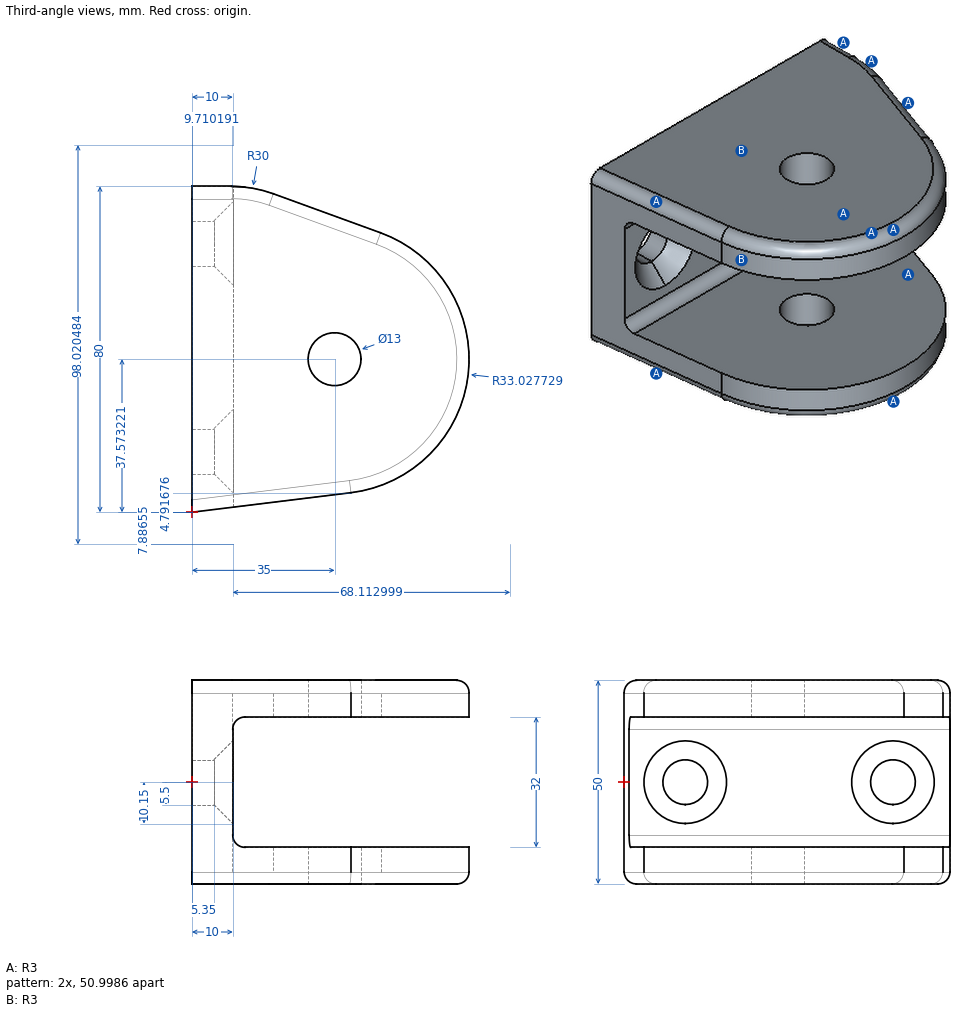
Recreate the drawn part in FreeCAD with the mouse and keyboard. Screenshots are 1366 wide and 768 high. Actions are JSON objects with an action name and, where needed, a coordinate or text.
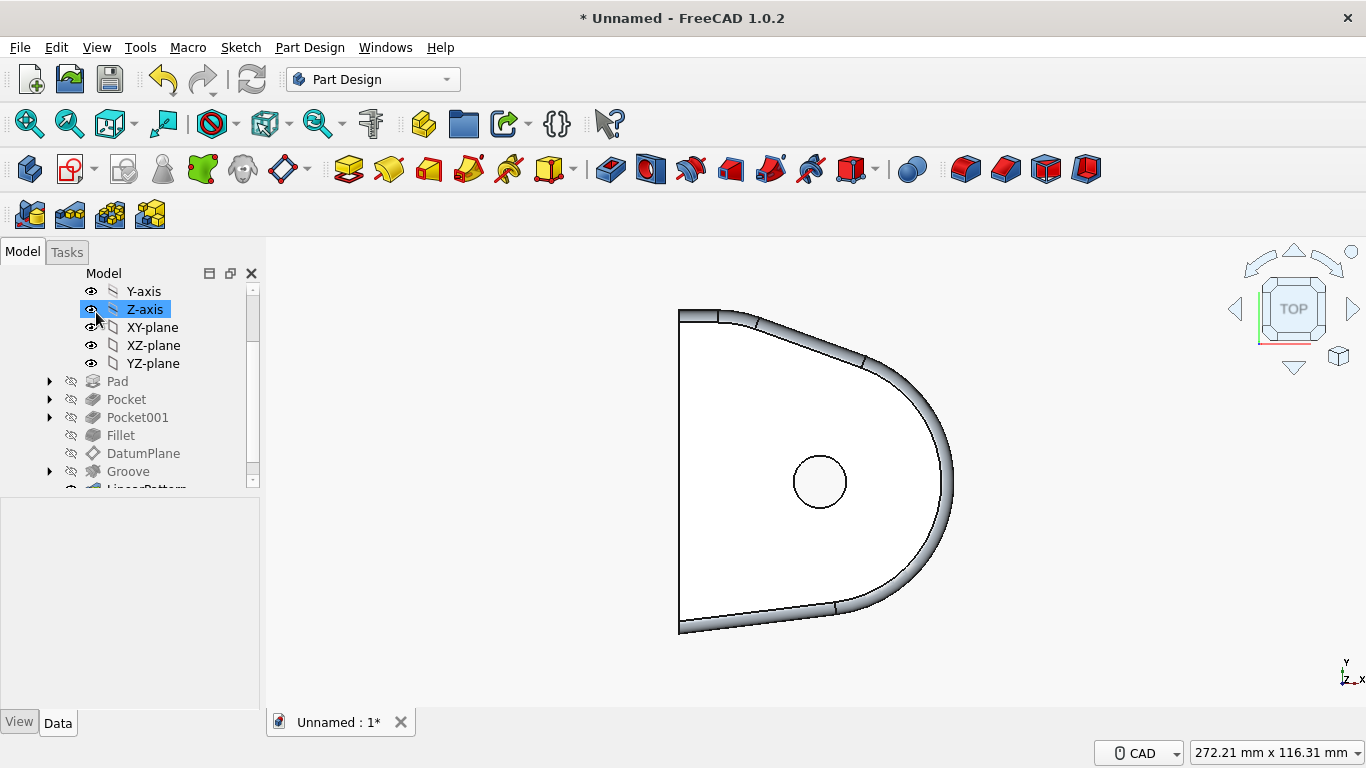
{"action": "key", "text": "1"}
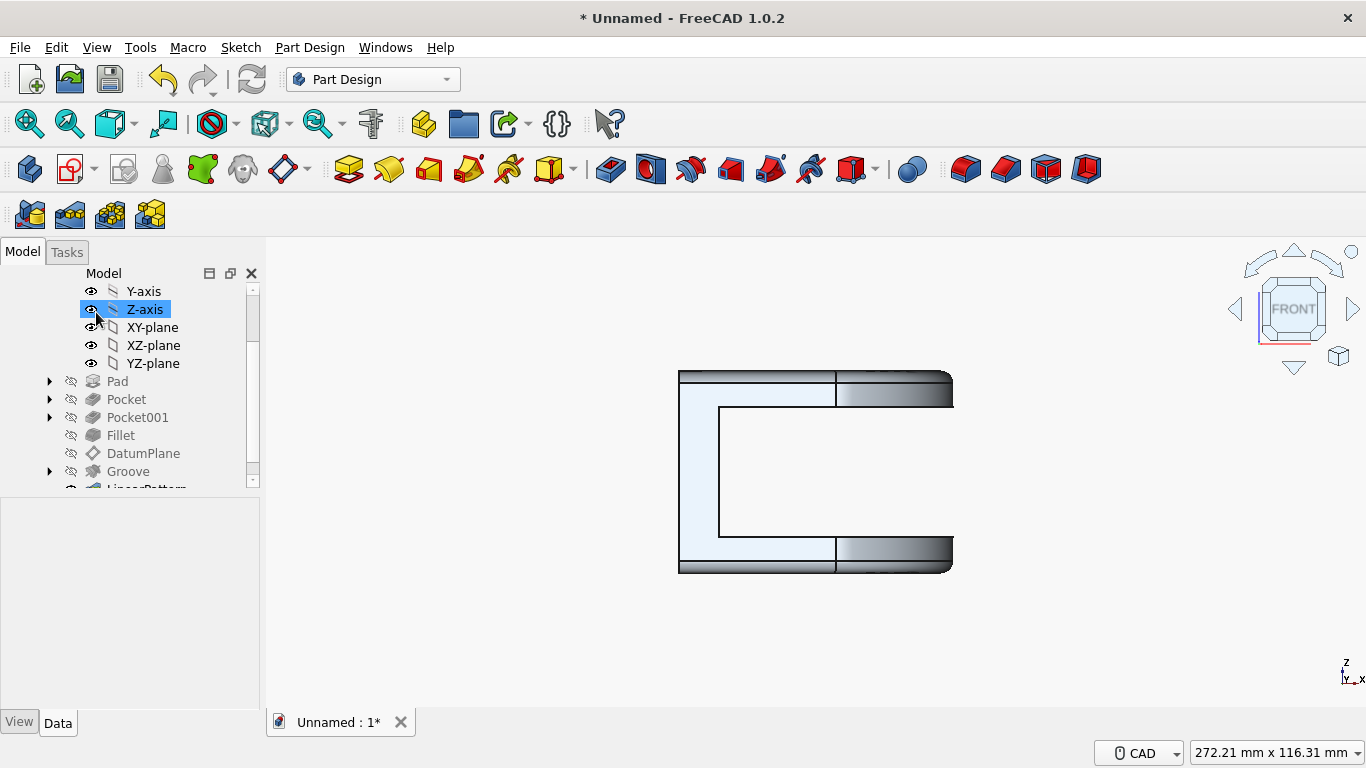
{"action": "left_click", "coordinate": [30, 124]}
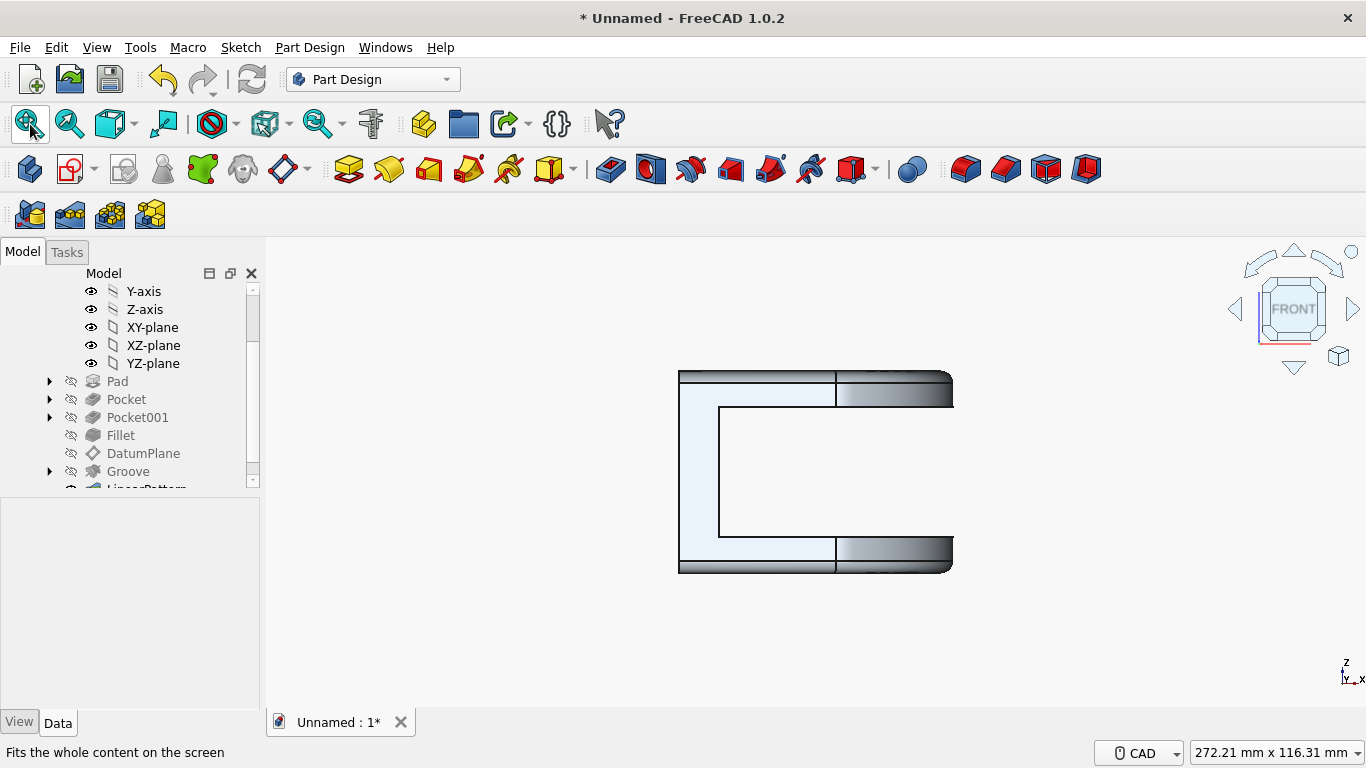
{"action": "key", "text": "3"}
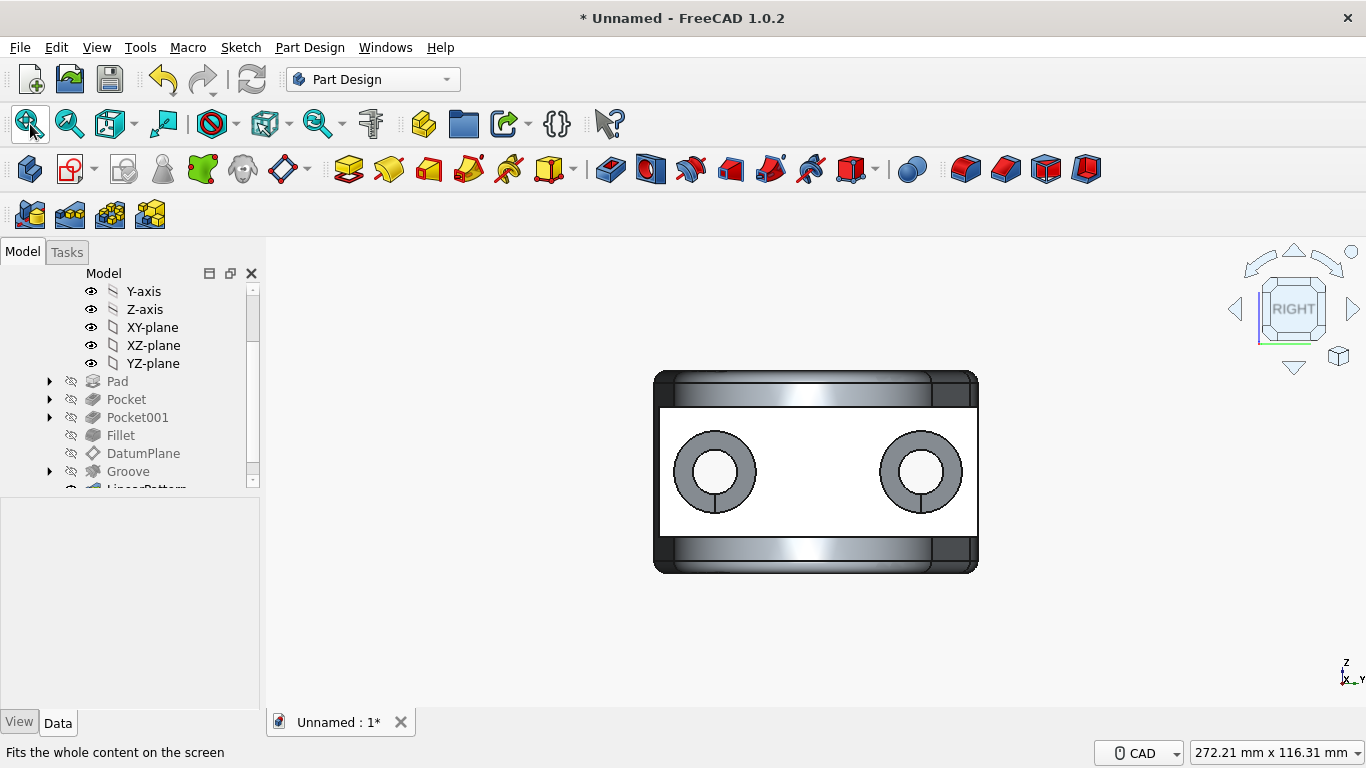
{"action": "left_click", "coordinate": [30, 124]}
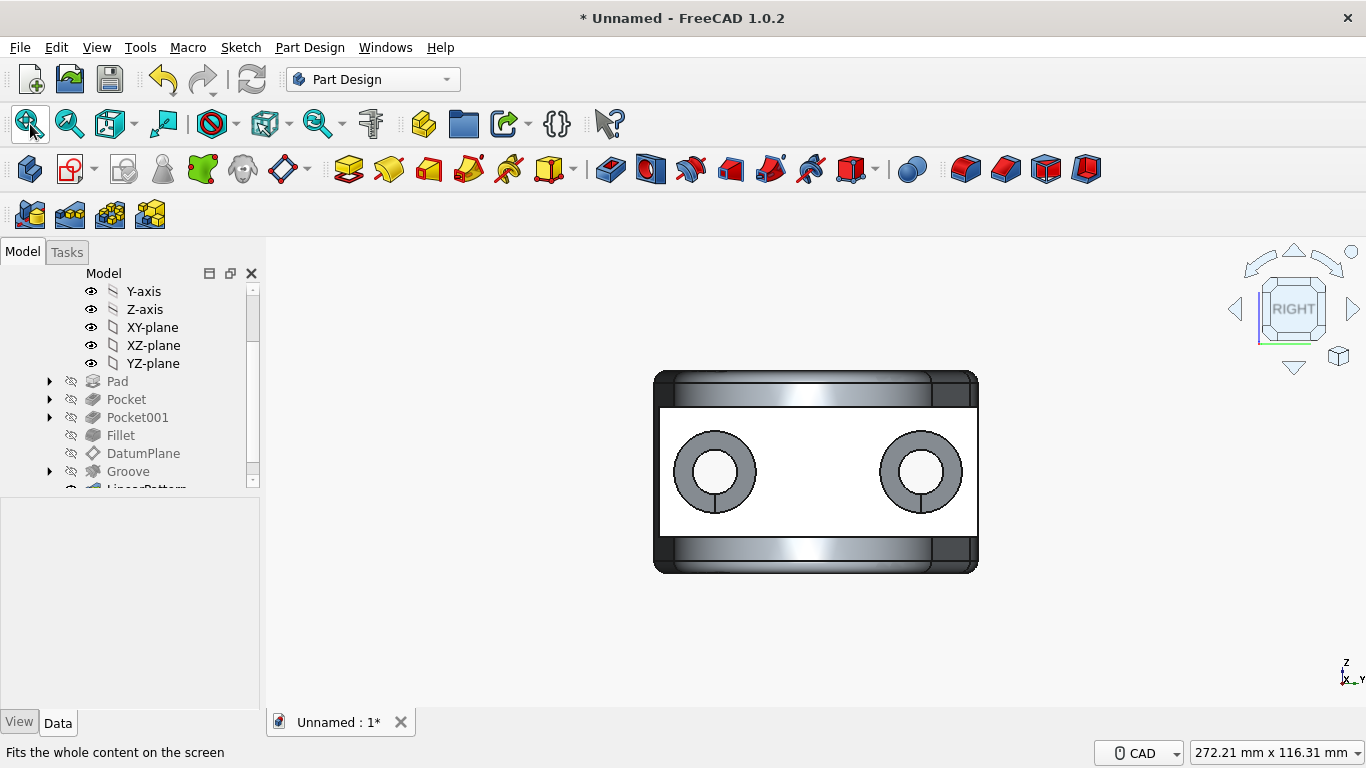
{"action": "key", "text": "5"}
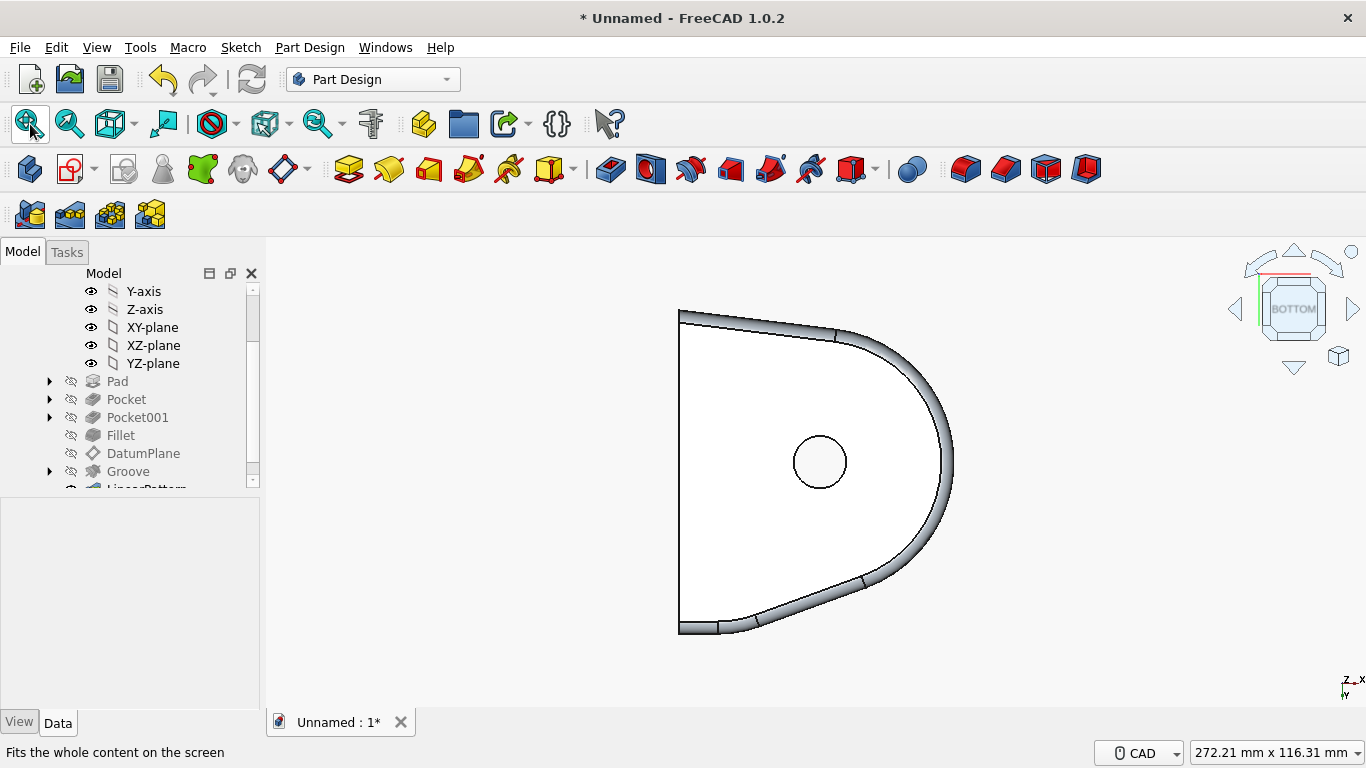
{"action": "key", "text": "4"}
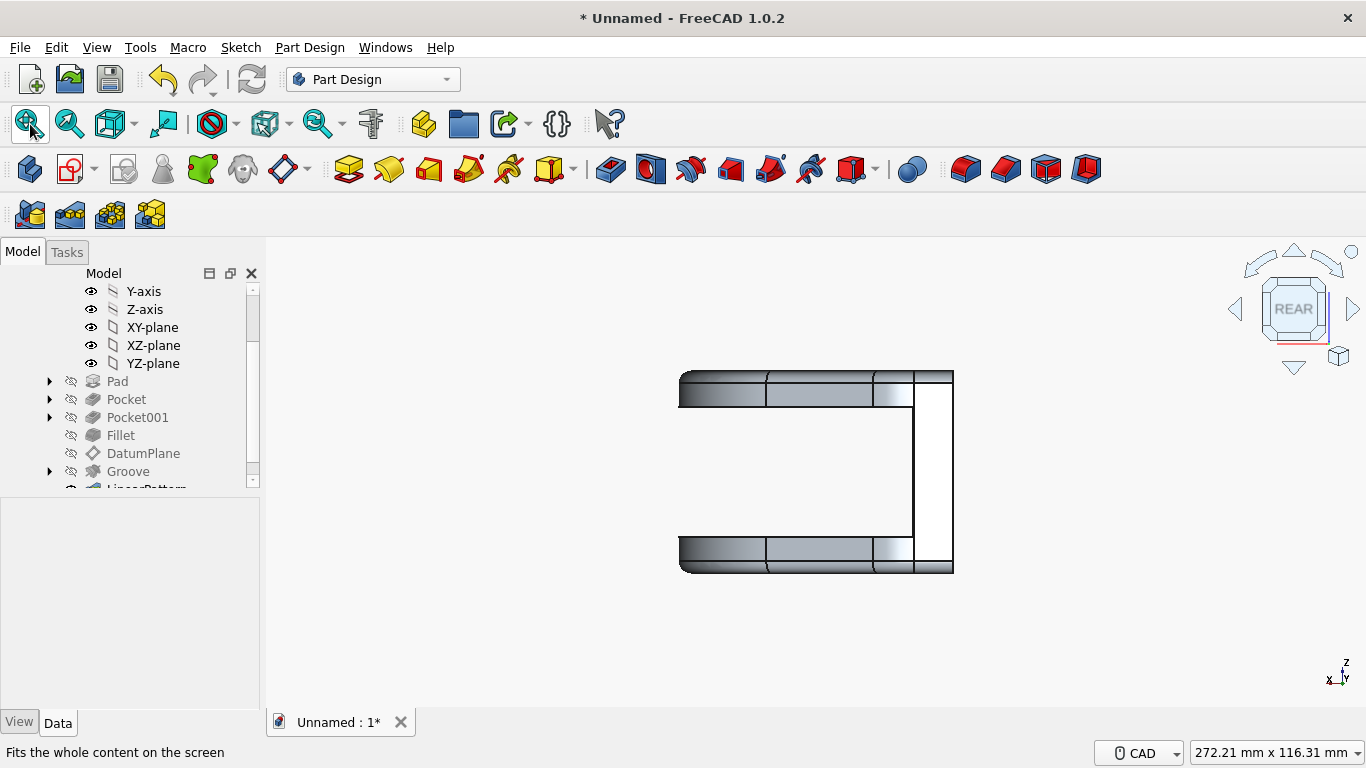
{"action": "left_click", "coordinate": [30, 124]}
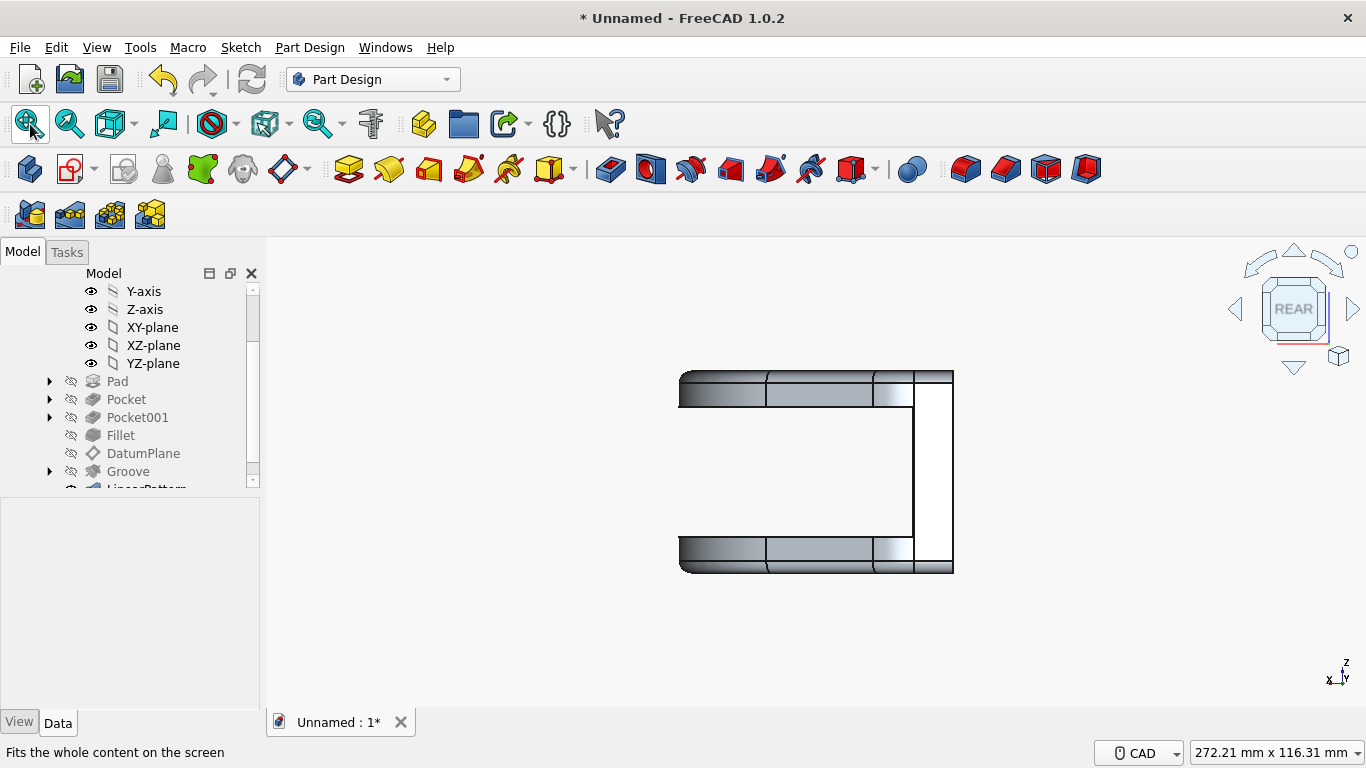
{"action": "key", "text": "6"}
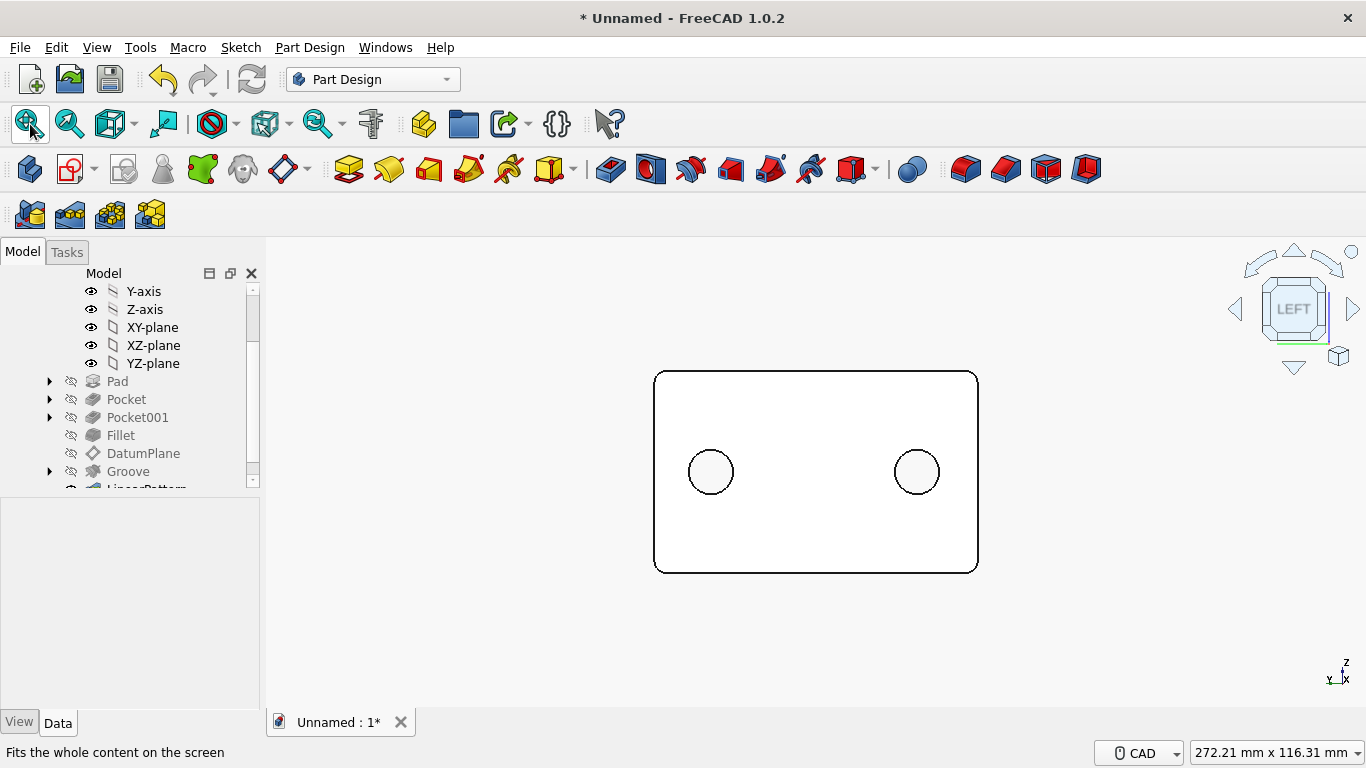
{"action": "left_click", "coordinate": [30, 124]}